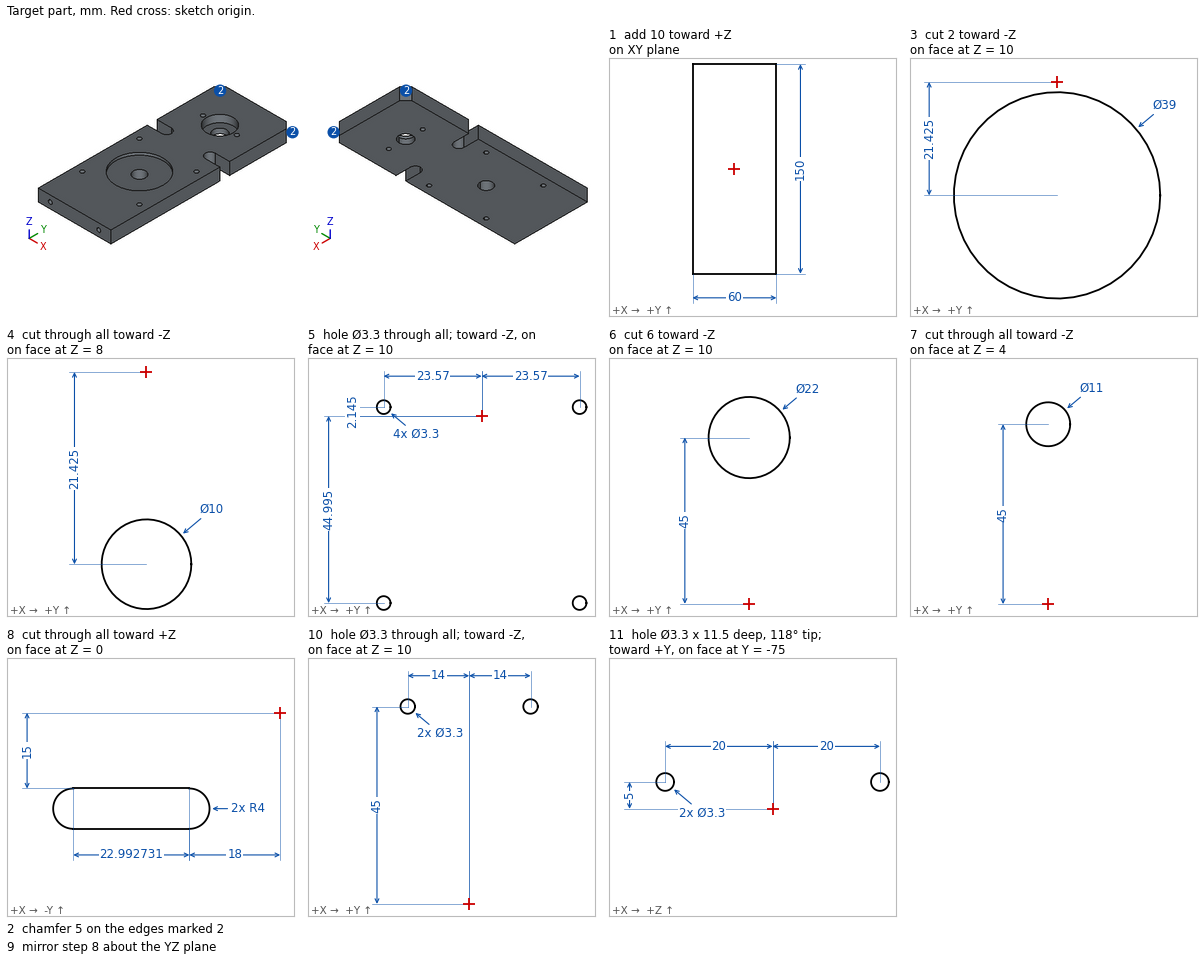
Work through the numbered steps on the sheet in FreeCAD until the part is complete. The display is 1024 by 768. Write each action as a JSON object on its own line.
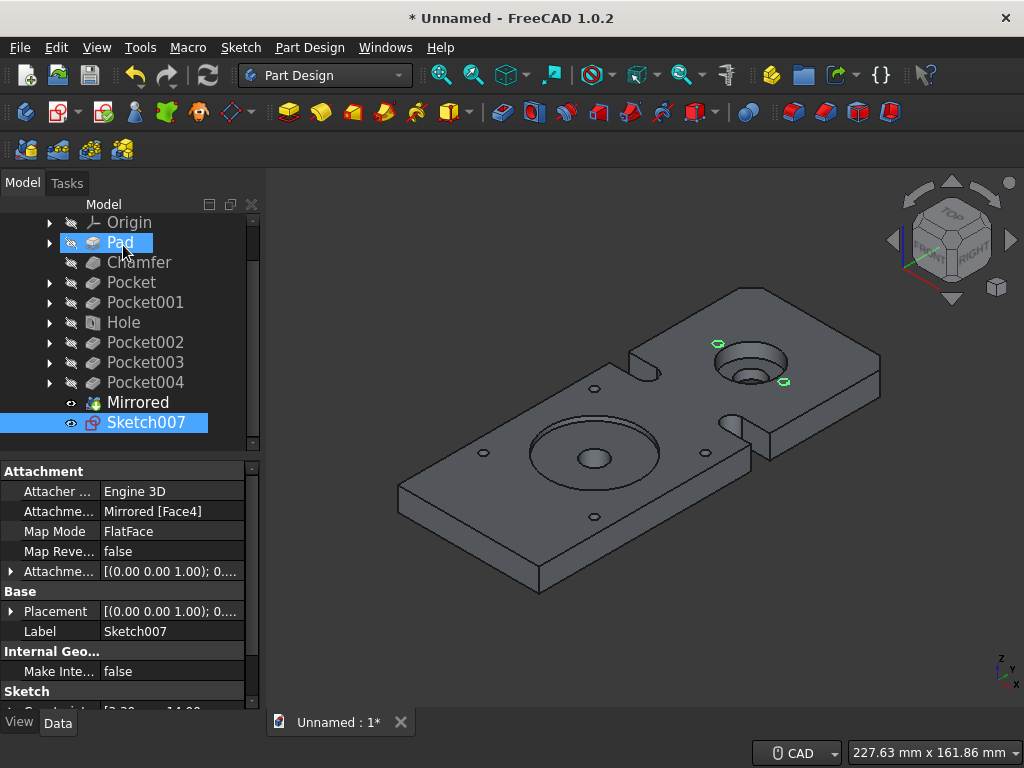
{"action": "left_click", "coordinate": [536, 112]}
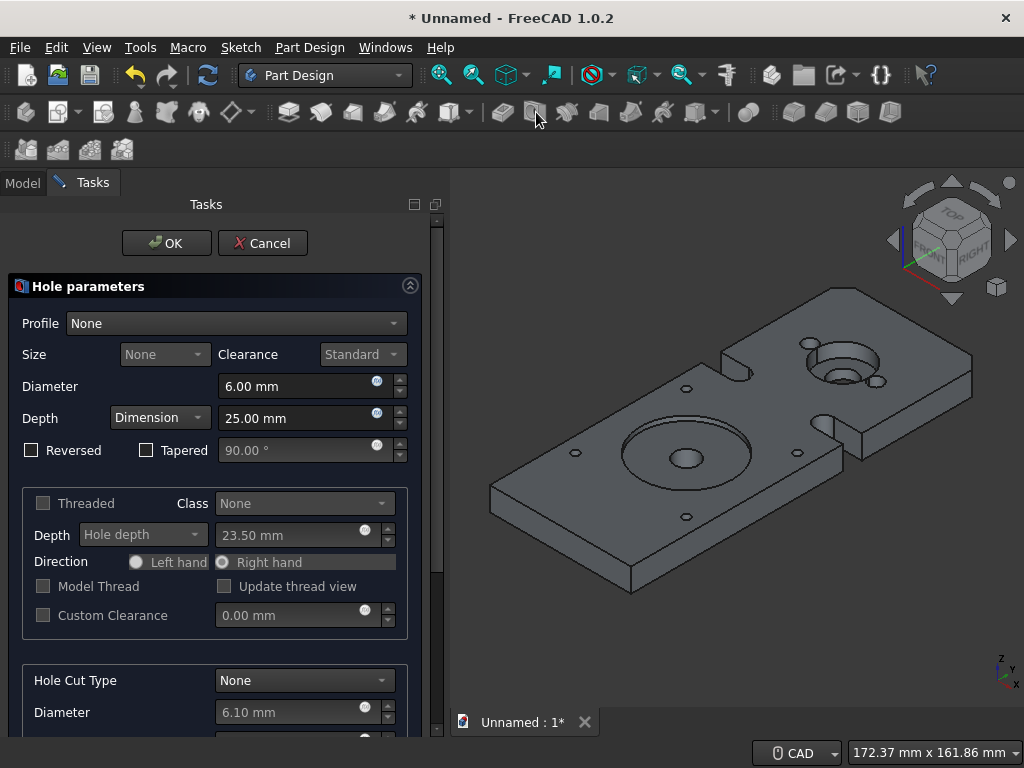
{"action": "triple_click", "coordinate": [305, 386]}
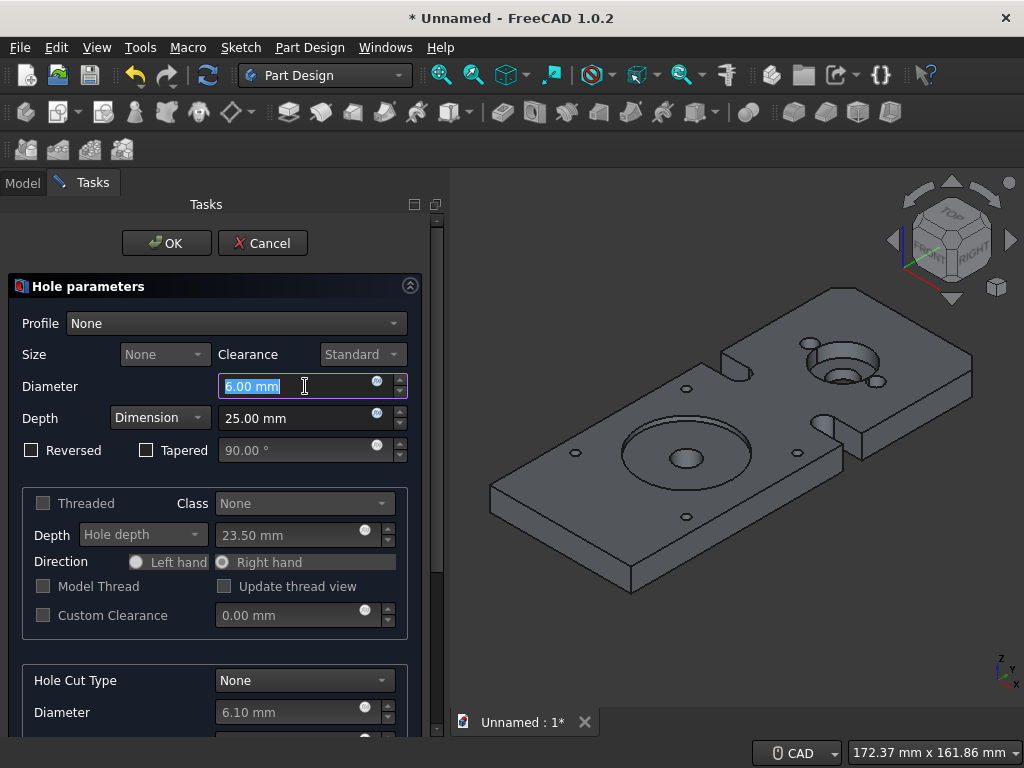
{"action": "type", "text": "3.3"}
{"action": "key", "text": "Tab"}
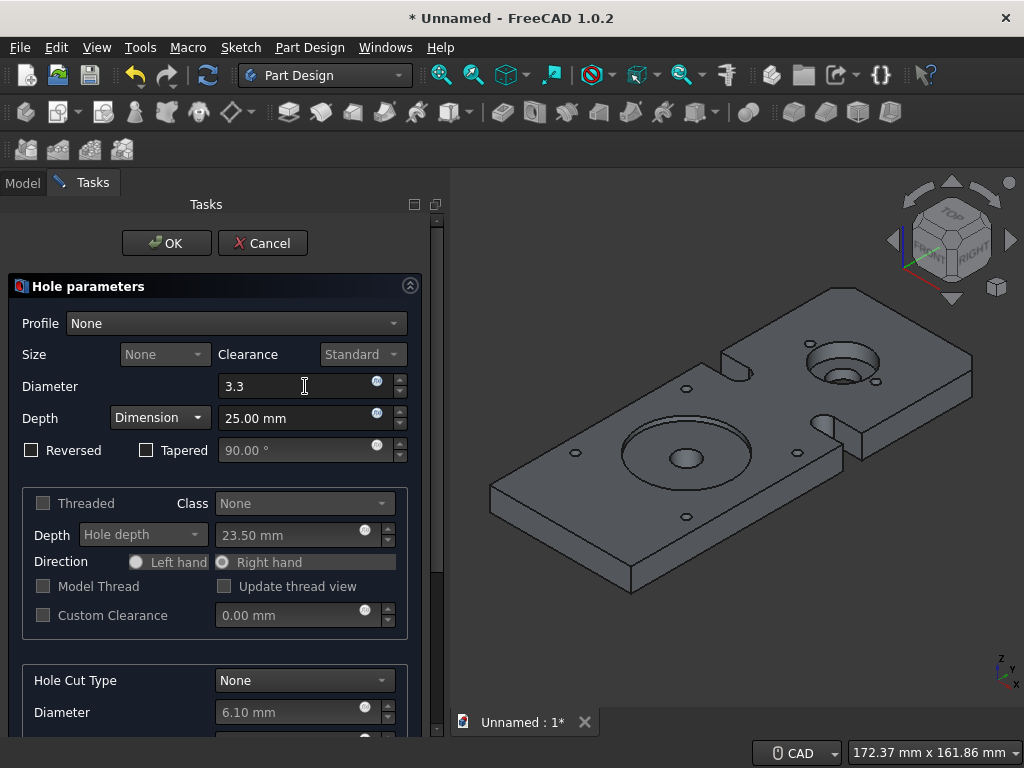
{"action": "left_click", "coordinate": [161, 418]}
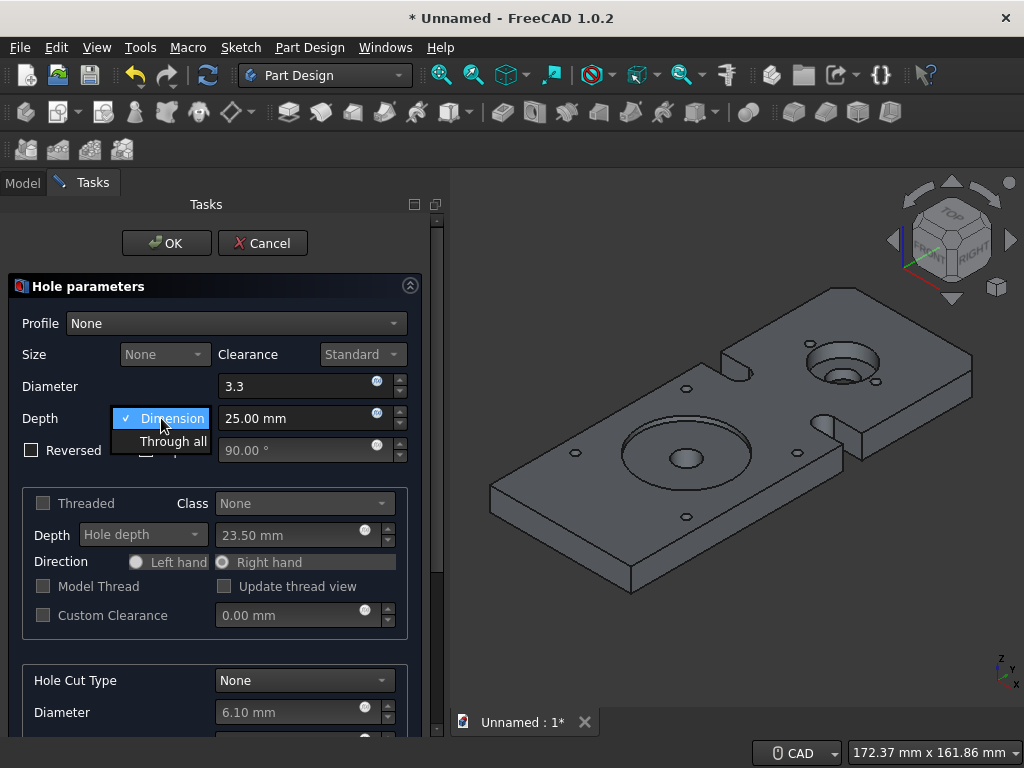
{"action": "left_click", "coordinate": [160, 442]}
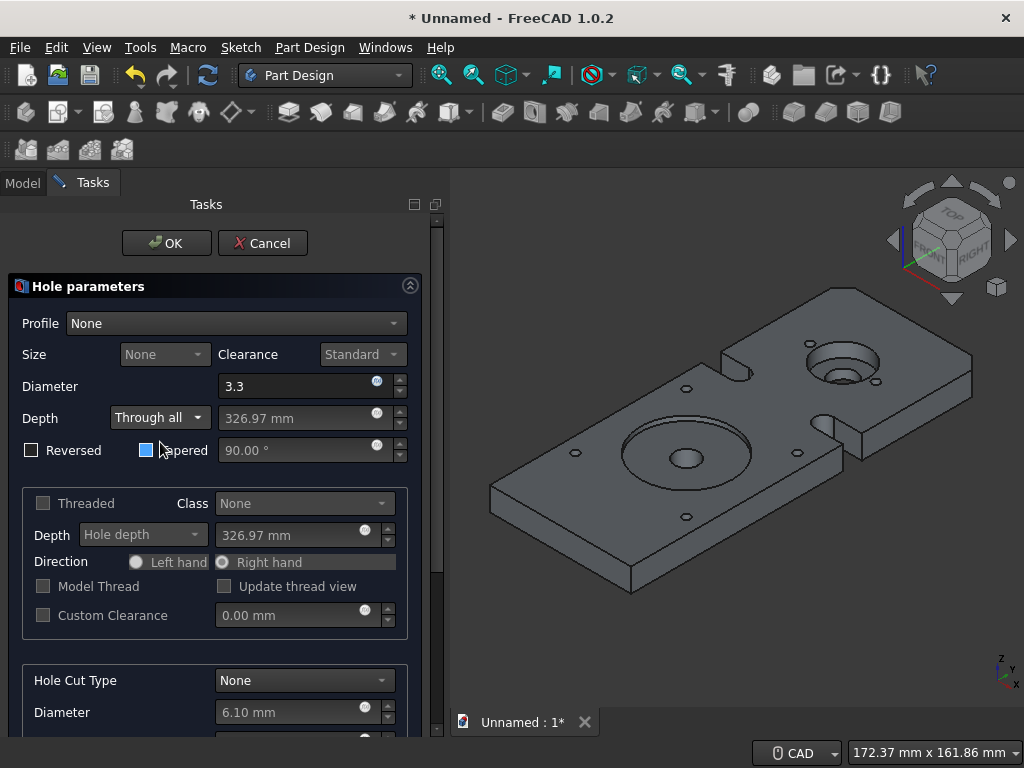
{"action": "left_click", "coordinate": [167, 243]}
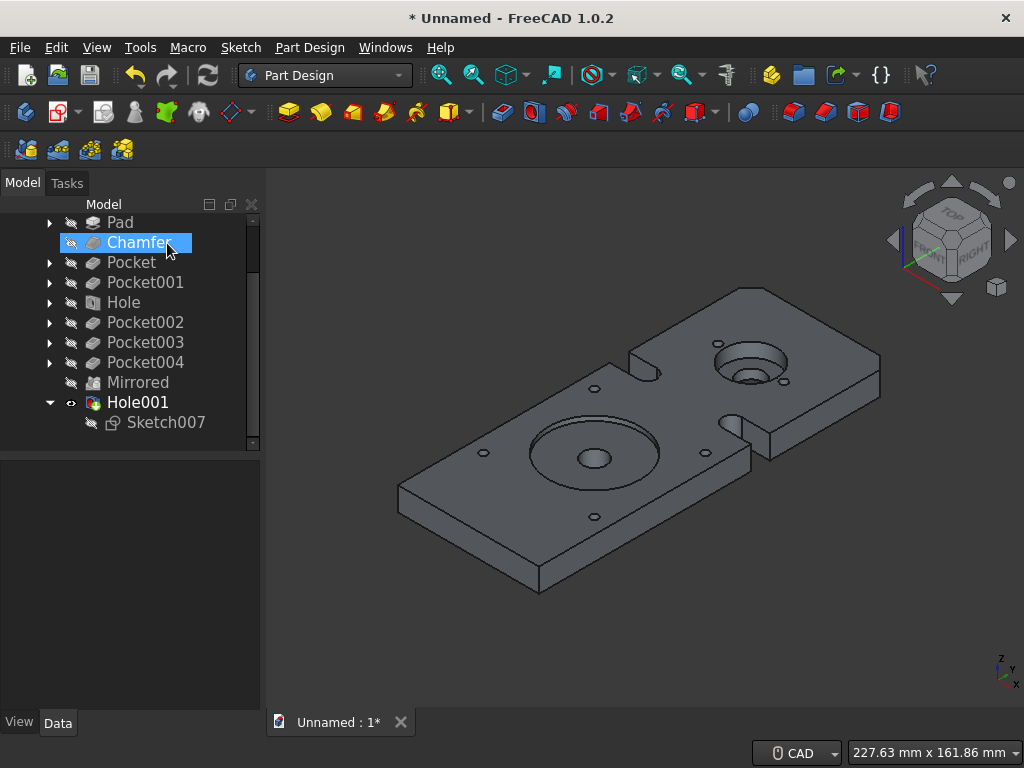
{"action": "left_click", "coordinate": [509, 562]}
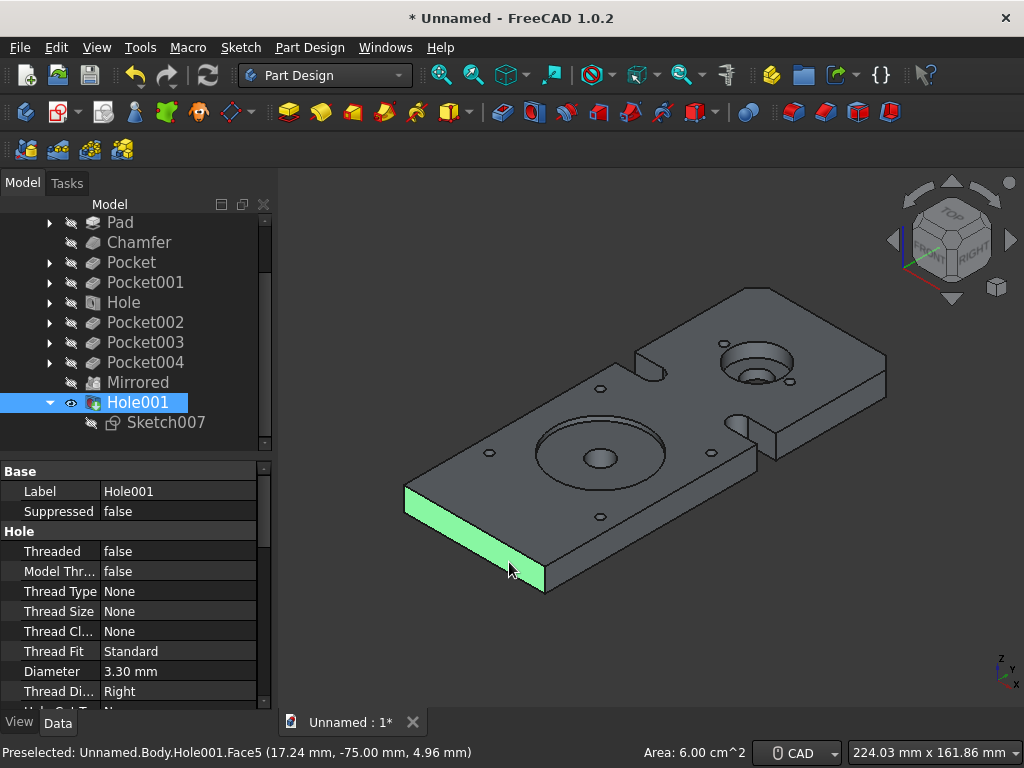
{"action": "left_click", "coordinate": [58, 112]}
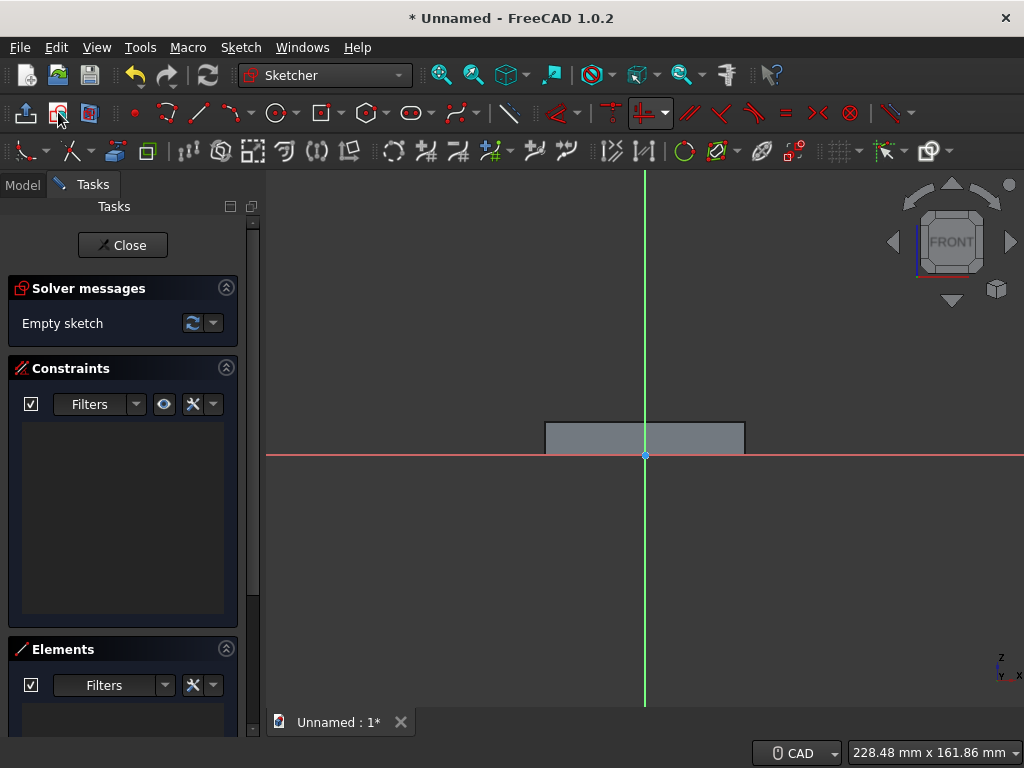
{"action": "scroll", "coordinate": [685, 447], "scroll_direction": "up", "scroll_amount": 5}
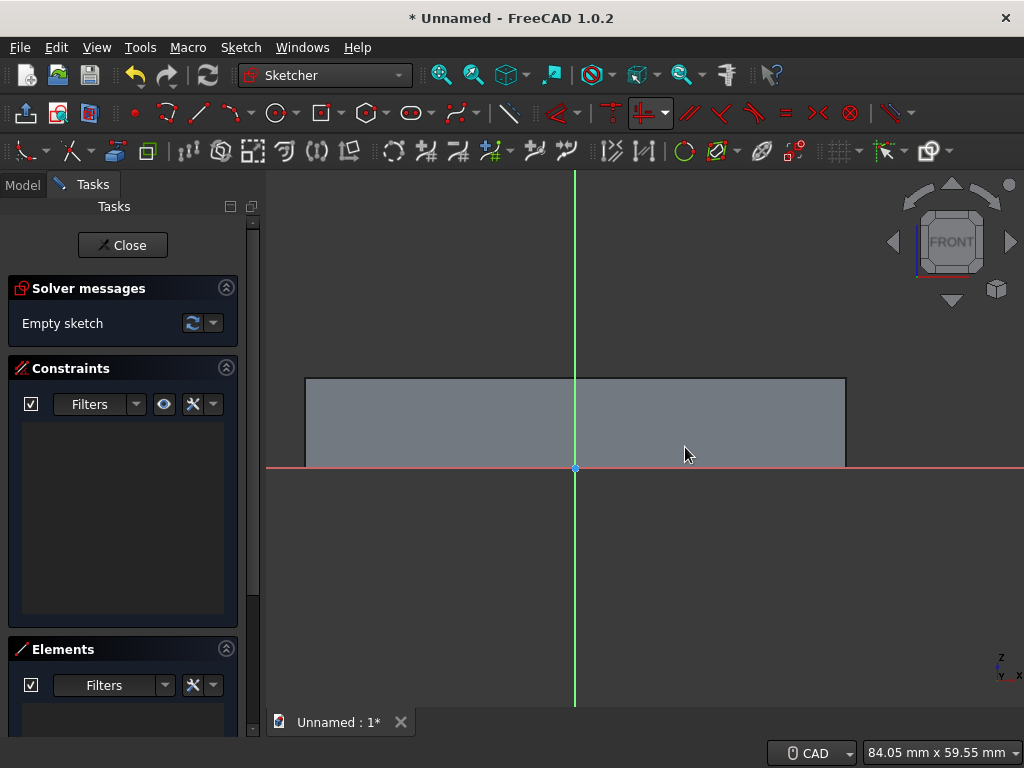
{"action": "key", "text": "g c"}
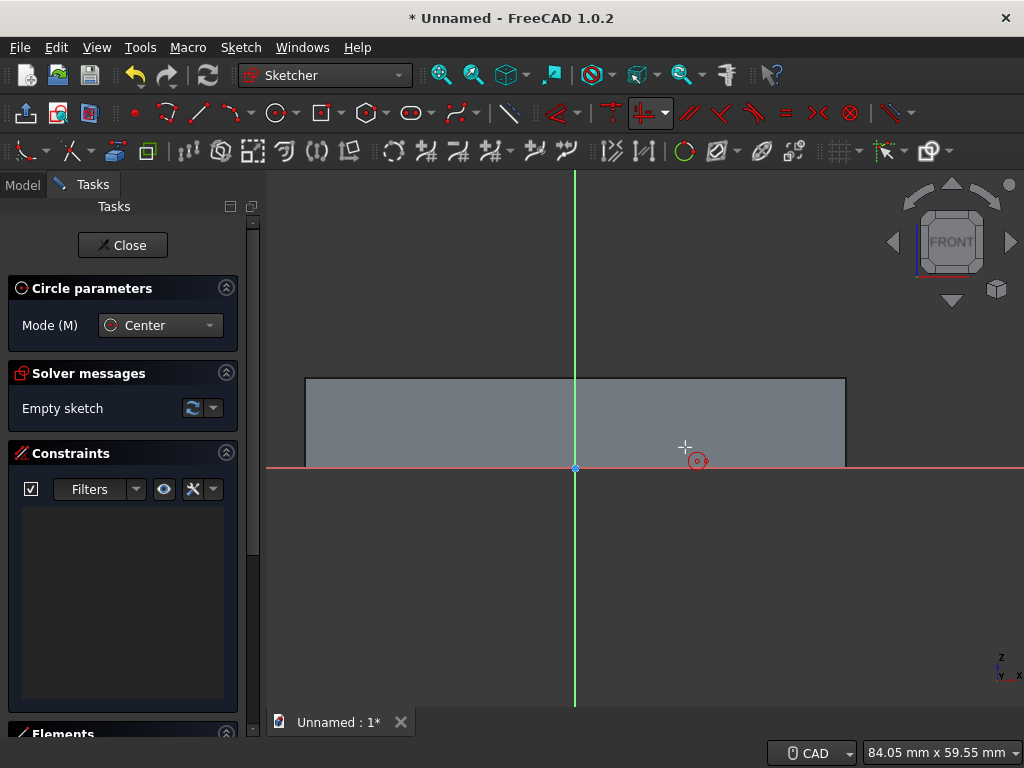
{"action": "scroll", "coordinate": [395, 423], "scroll_direction": "up", "scroll_amount": 3}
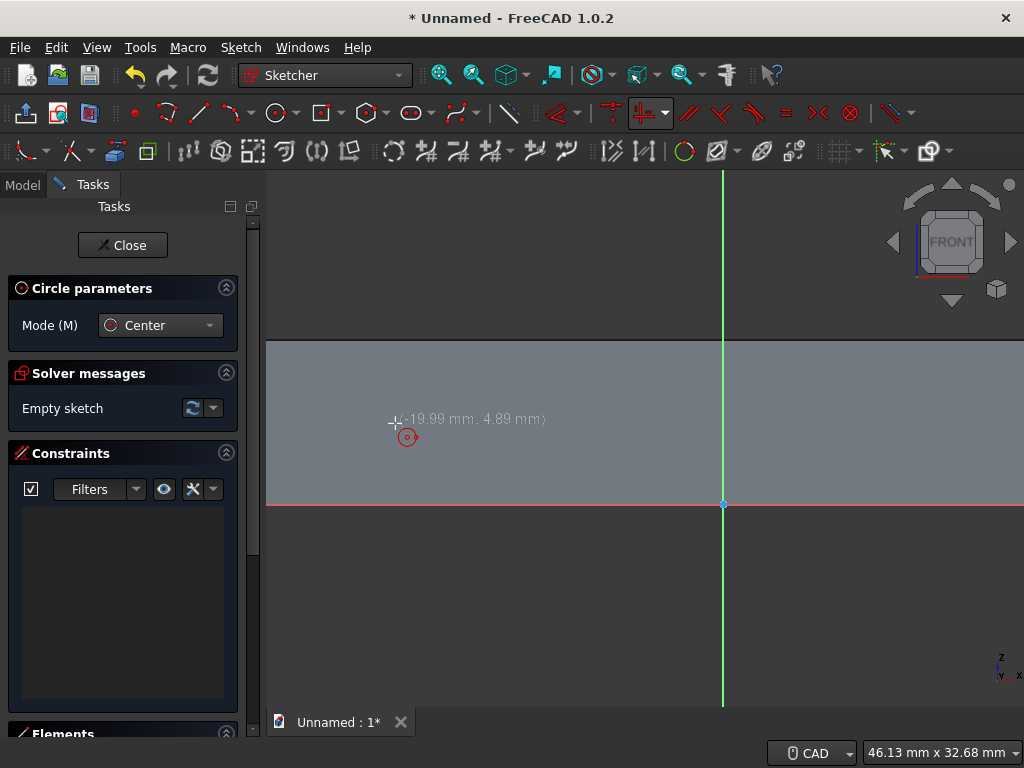
{"action": "left_click", "coordinate": [395, 423]}
{"action": "left_click", "coordinate": [414, 403]}